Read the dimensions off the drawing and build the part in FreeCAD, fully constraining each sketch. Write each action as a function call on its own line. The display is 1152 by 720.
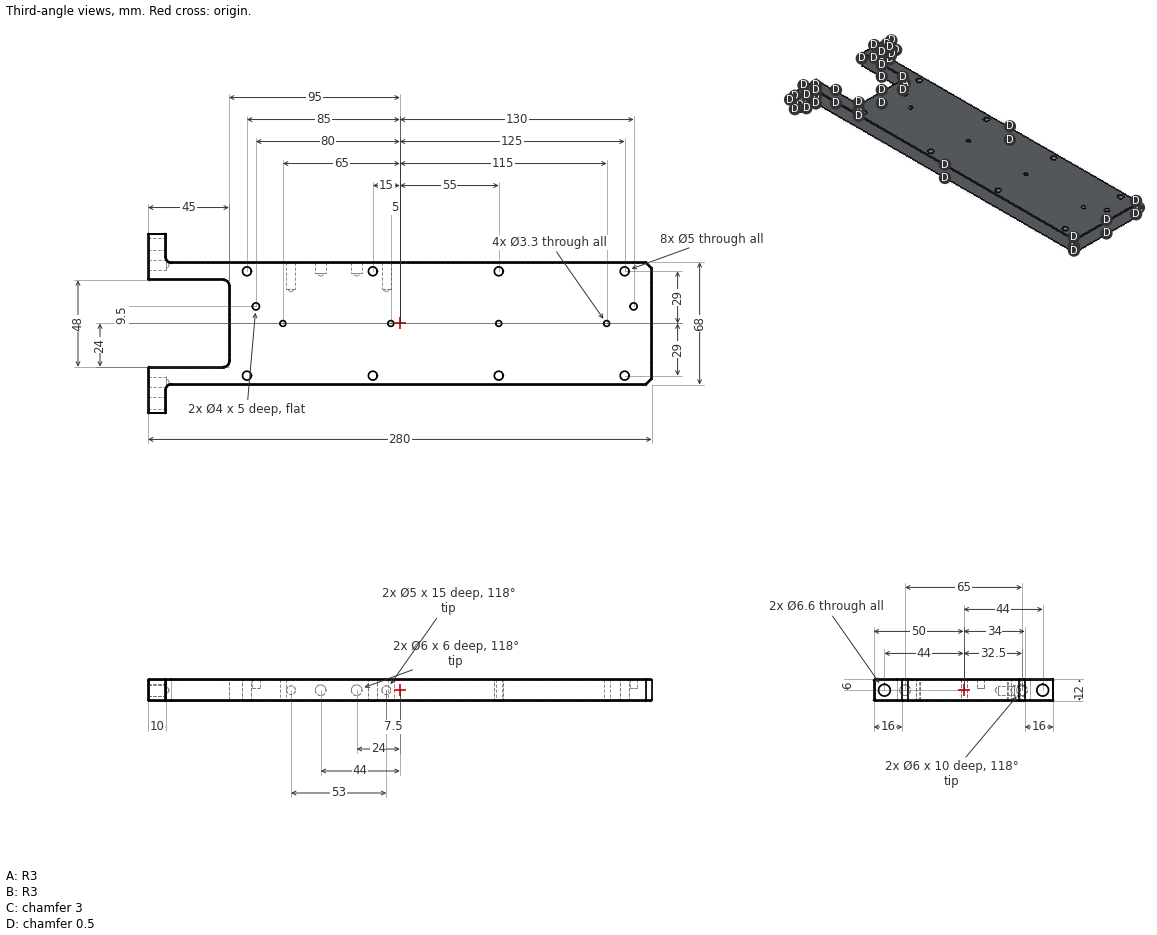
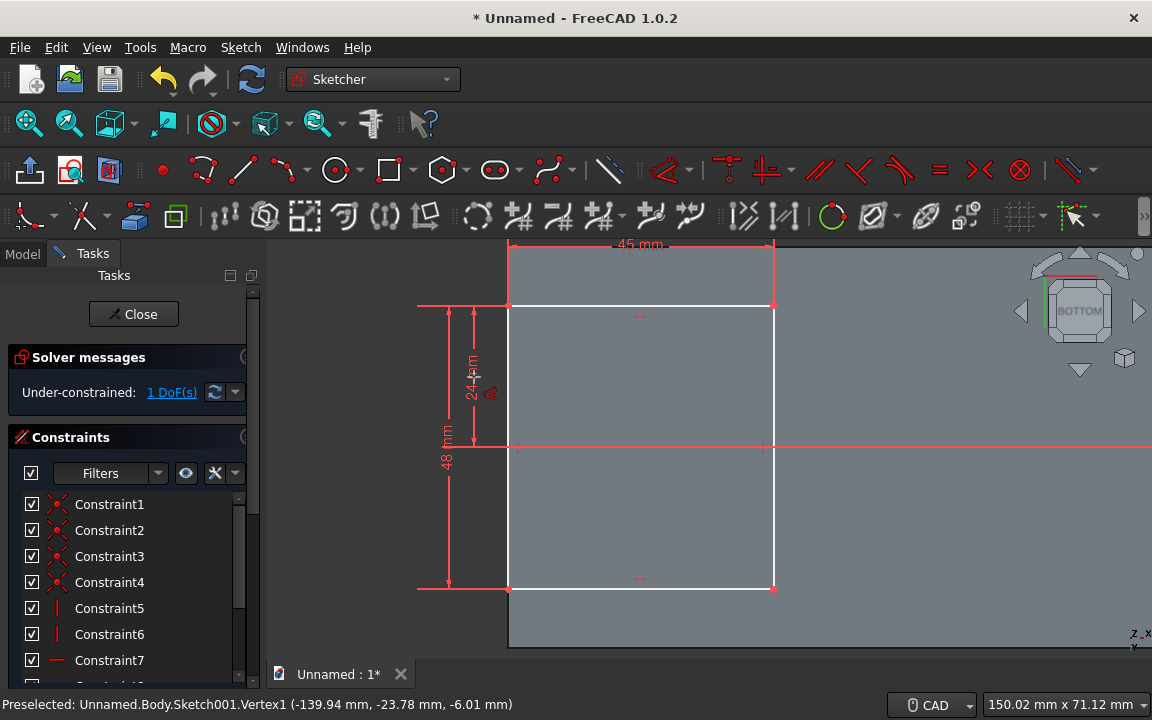
click(774, 589)
click(880, 623)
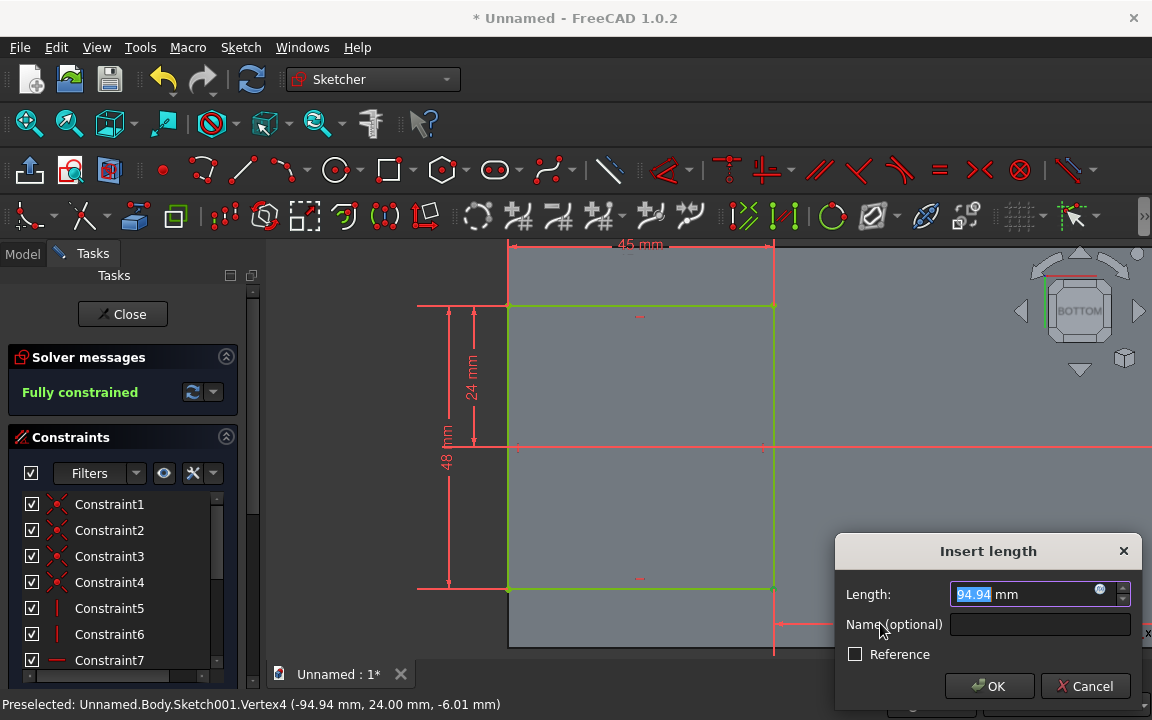
text(95)
key(Return)
key(Escape)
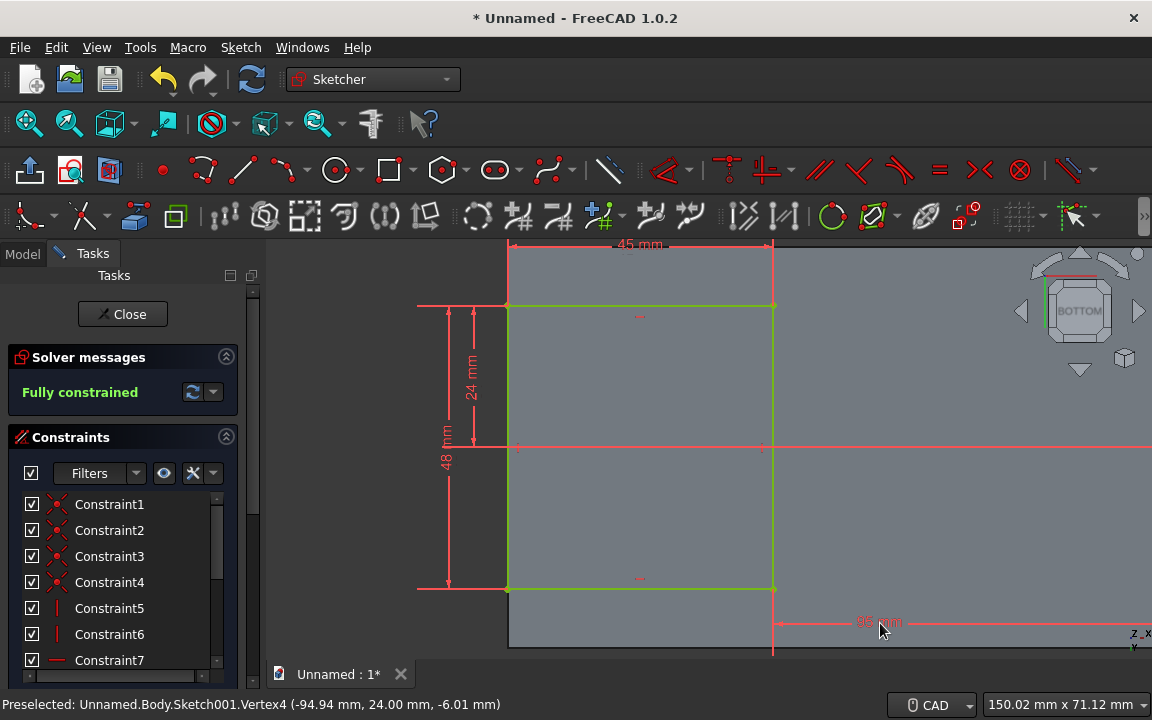
click(123, 314)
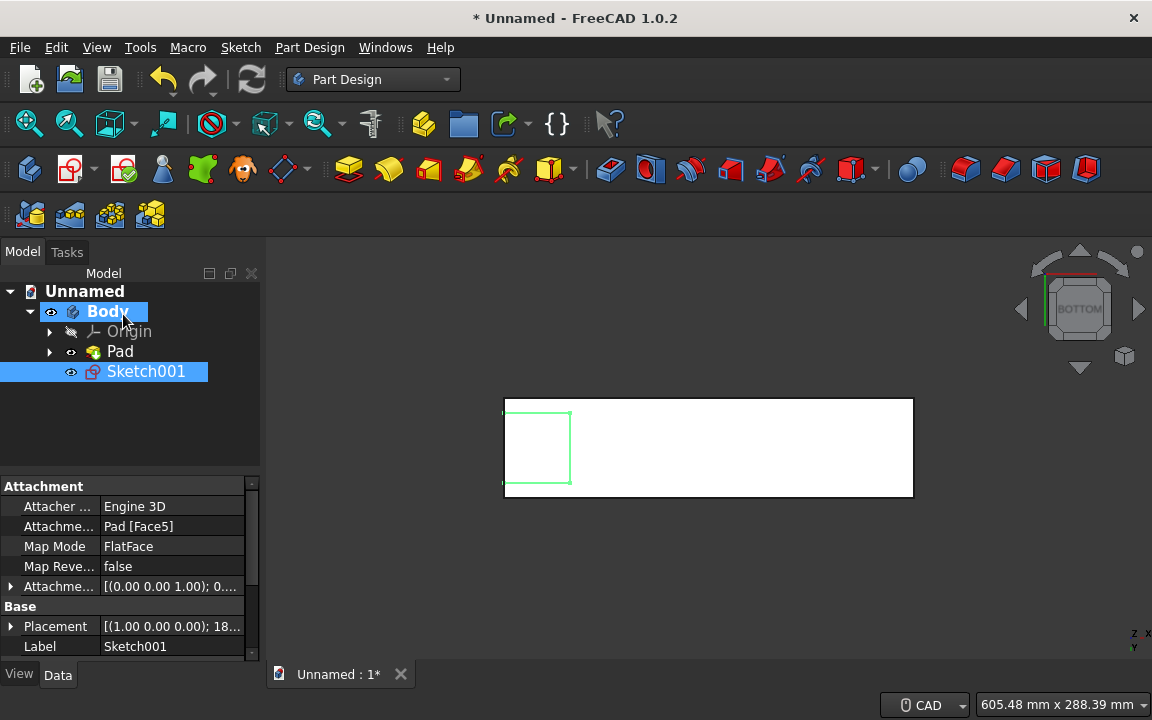
click(612, 170)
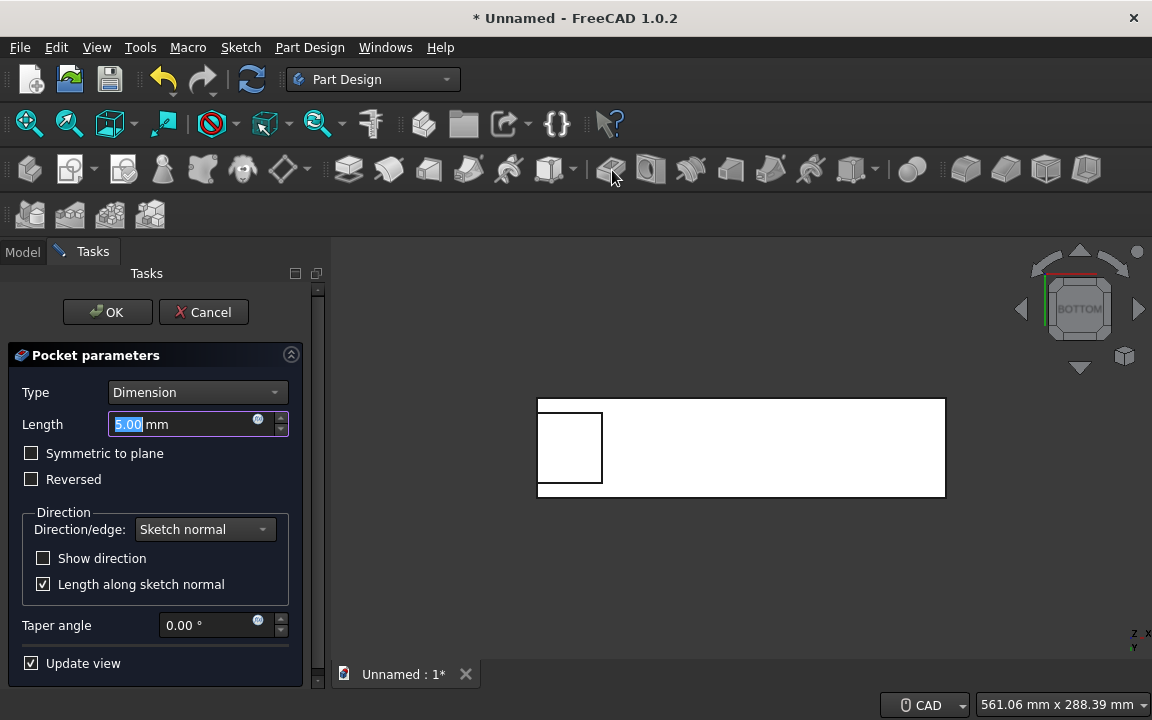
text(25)
key(Tab)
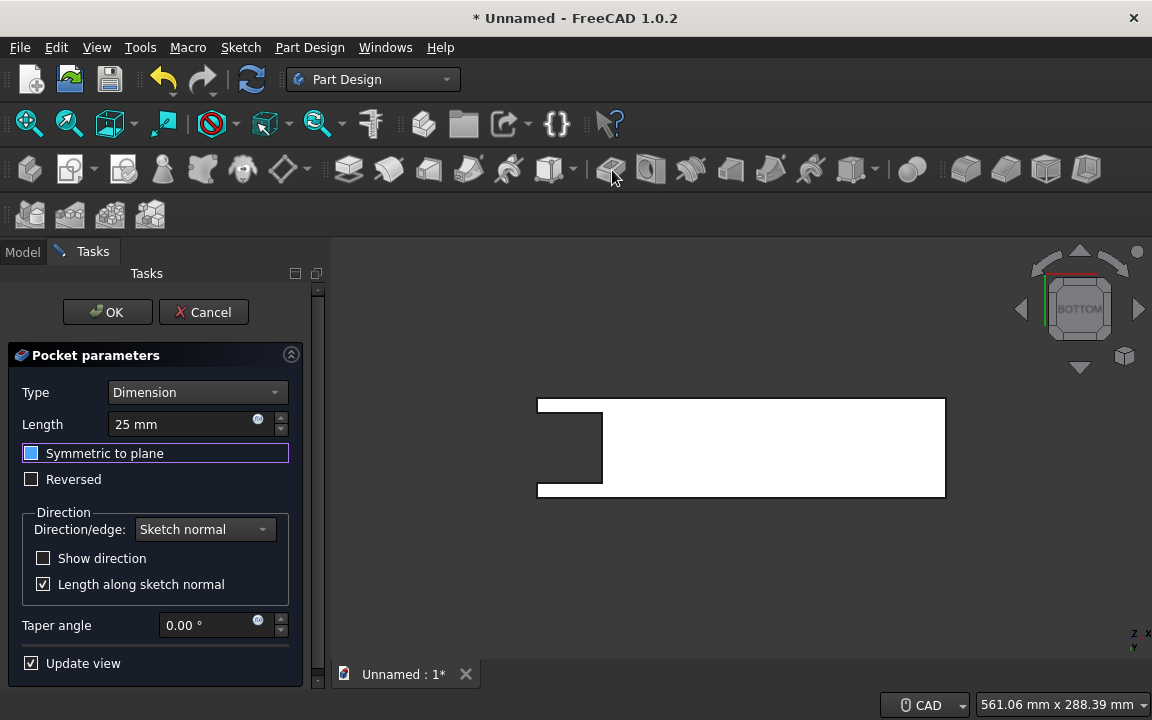
click(108, 312)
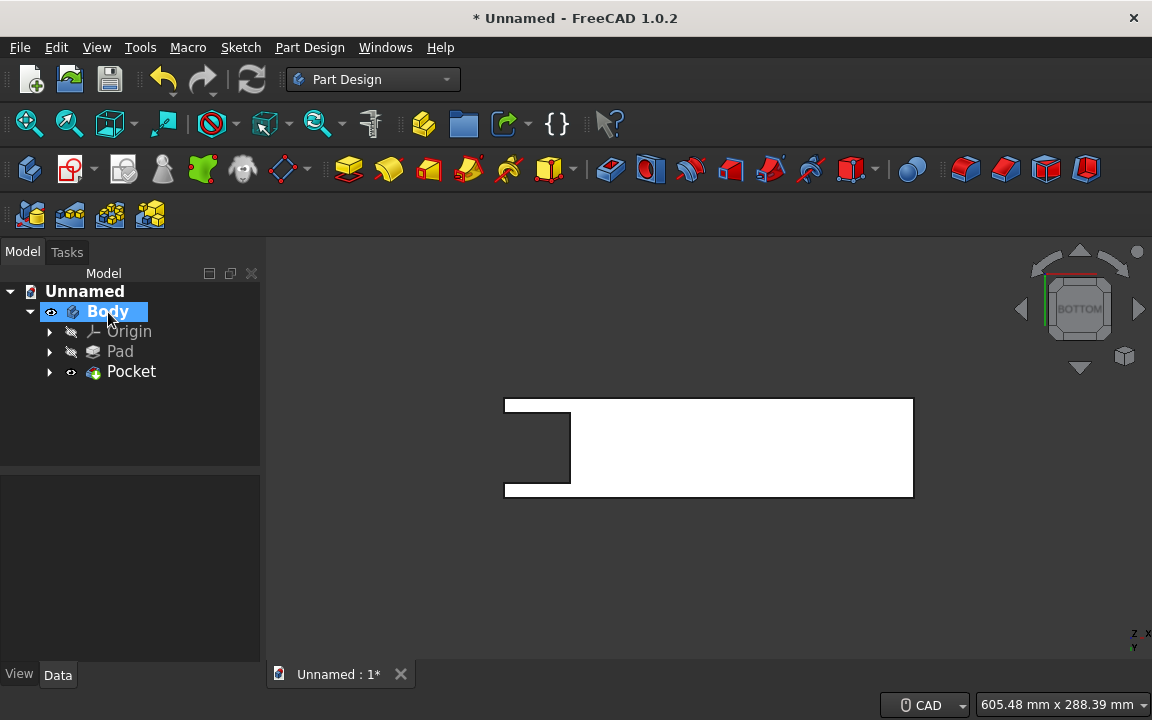
scroll(570, 412, up, 5)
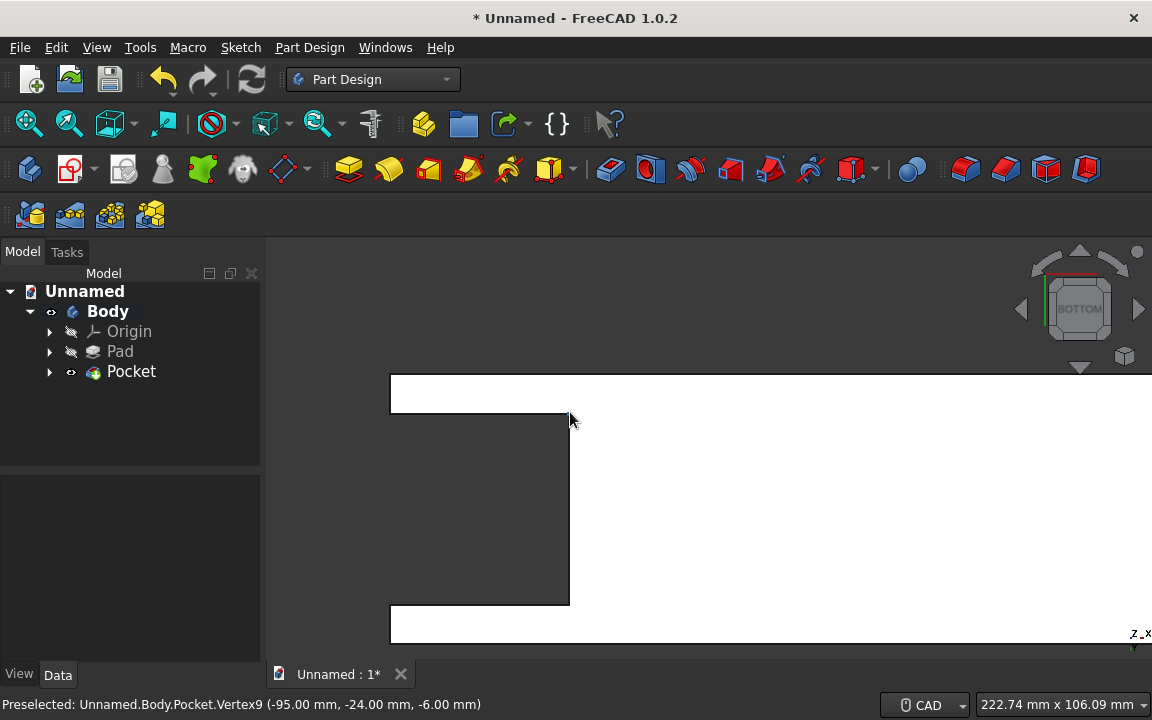
key(v)
key(f)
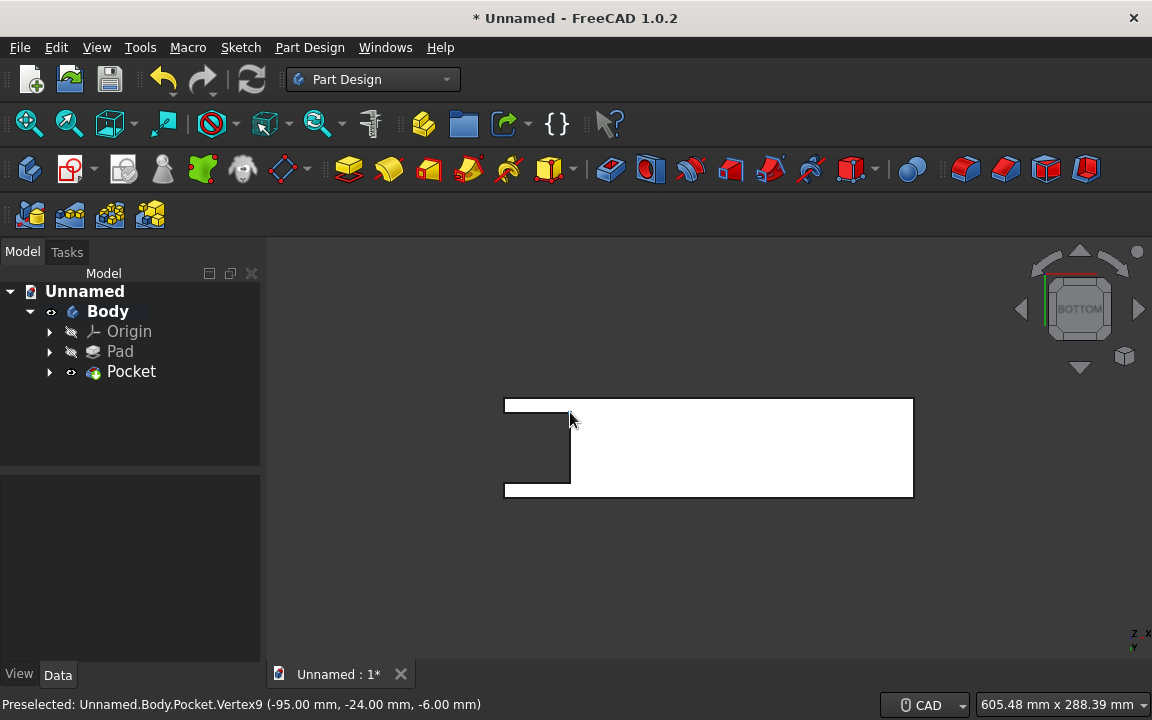
key(0)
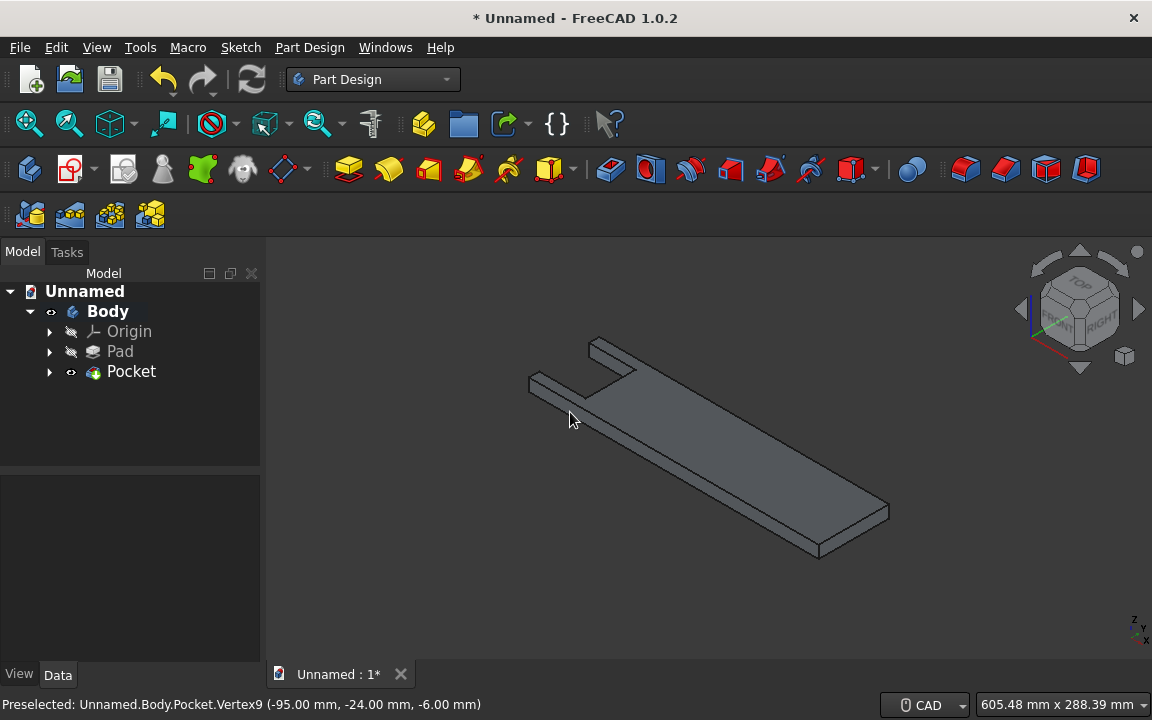
scroll(586, 405, up, 5)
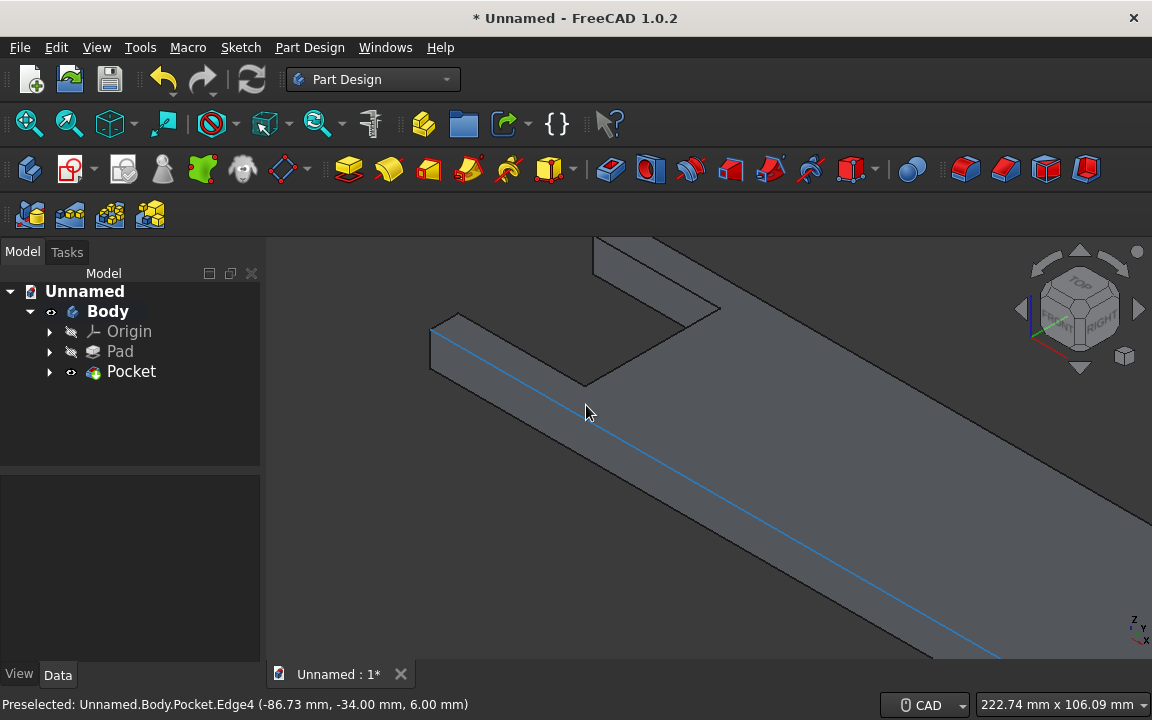
key(v)
key(f)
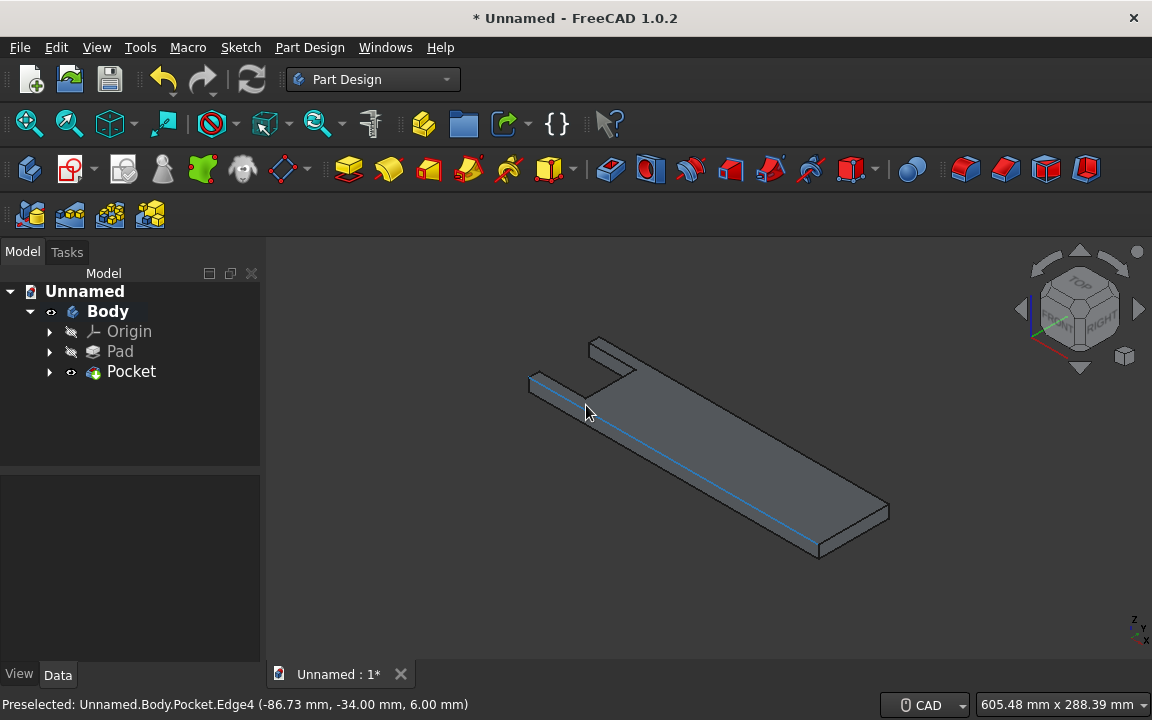
key(2)